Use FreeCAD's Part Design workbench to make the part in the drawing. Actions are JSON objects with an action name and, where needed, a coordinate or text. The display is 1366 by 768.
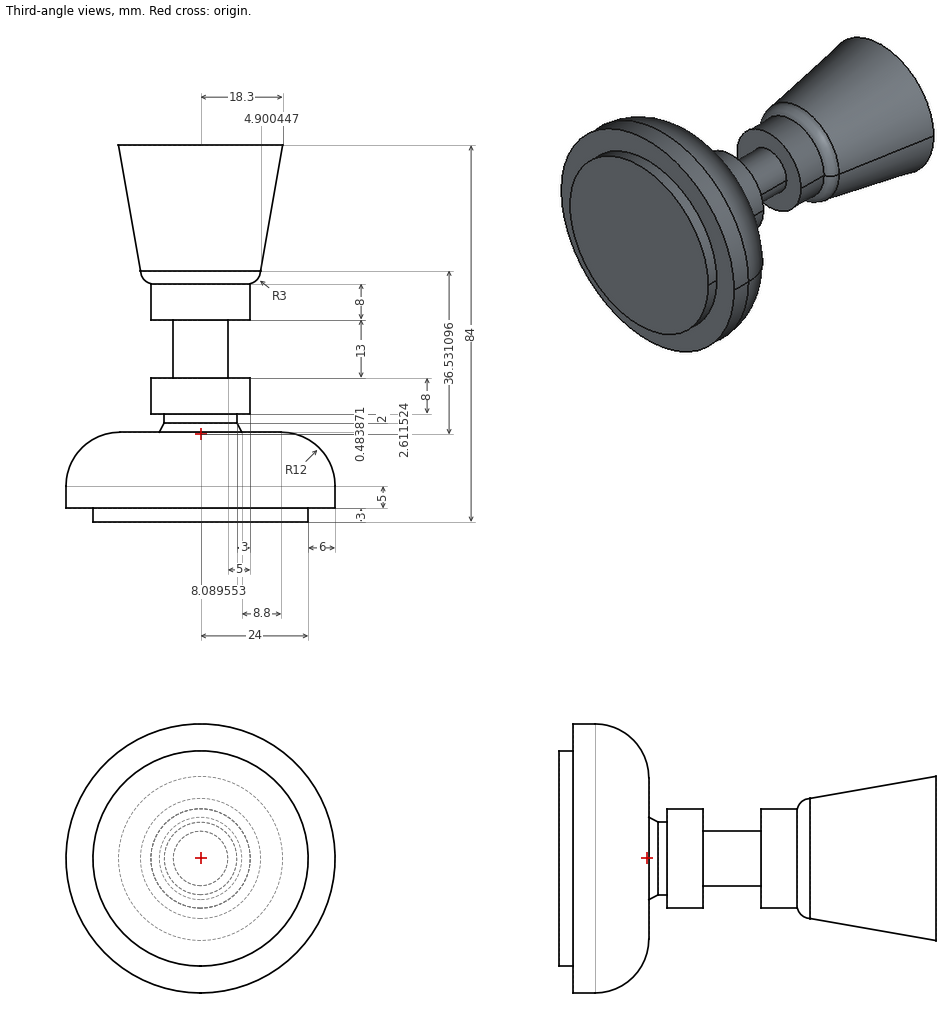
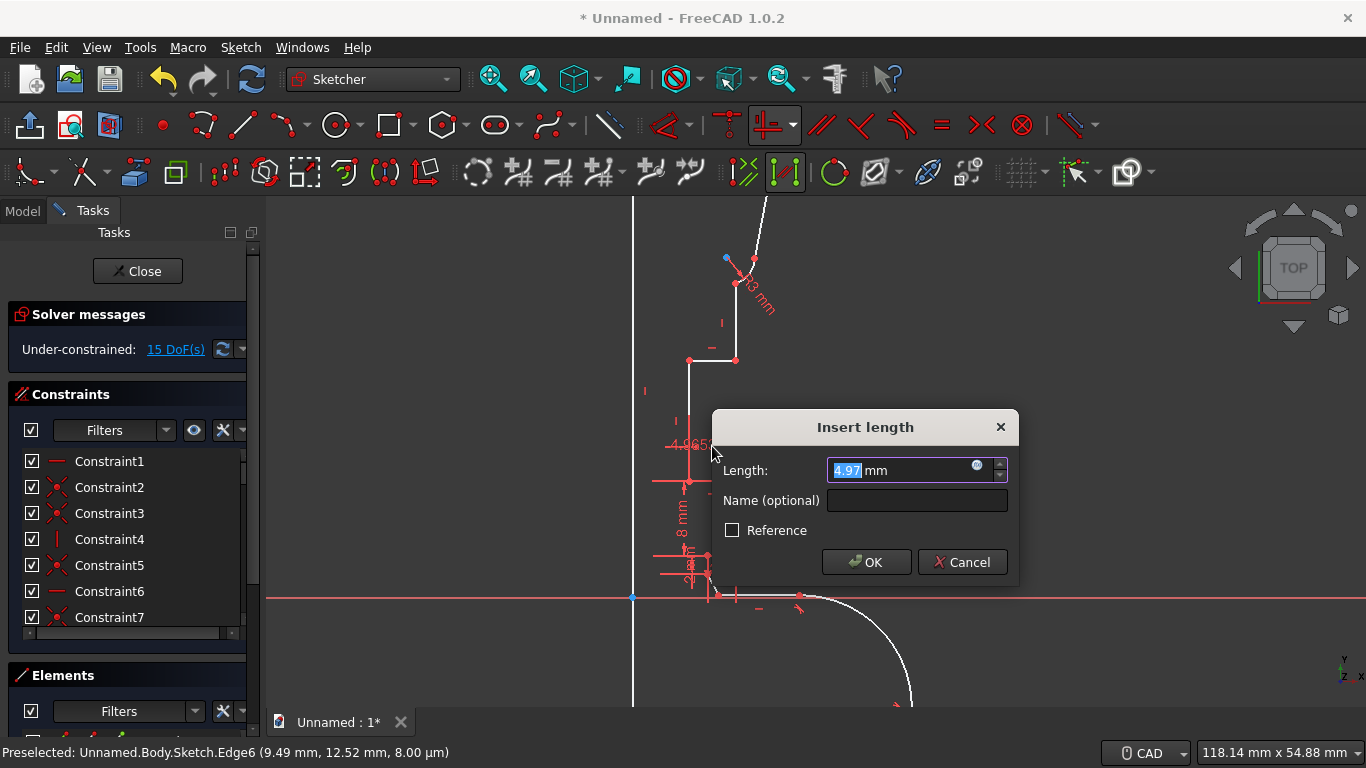
{"action": "type", "text": "5"}
{"action": "key", "text": "Return"}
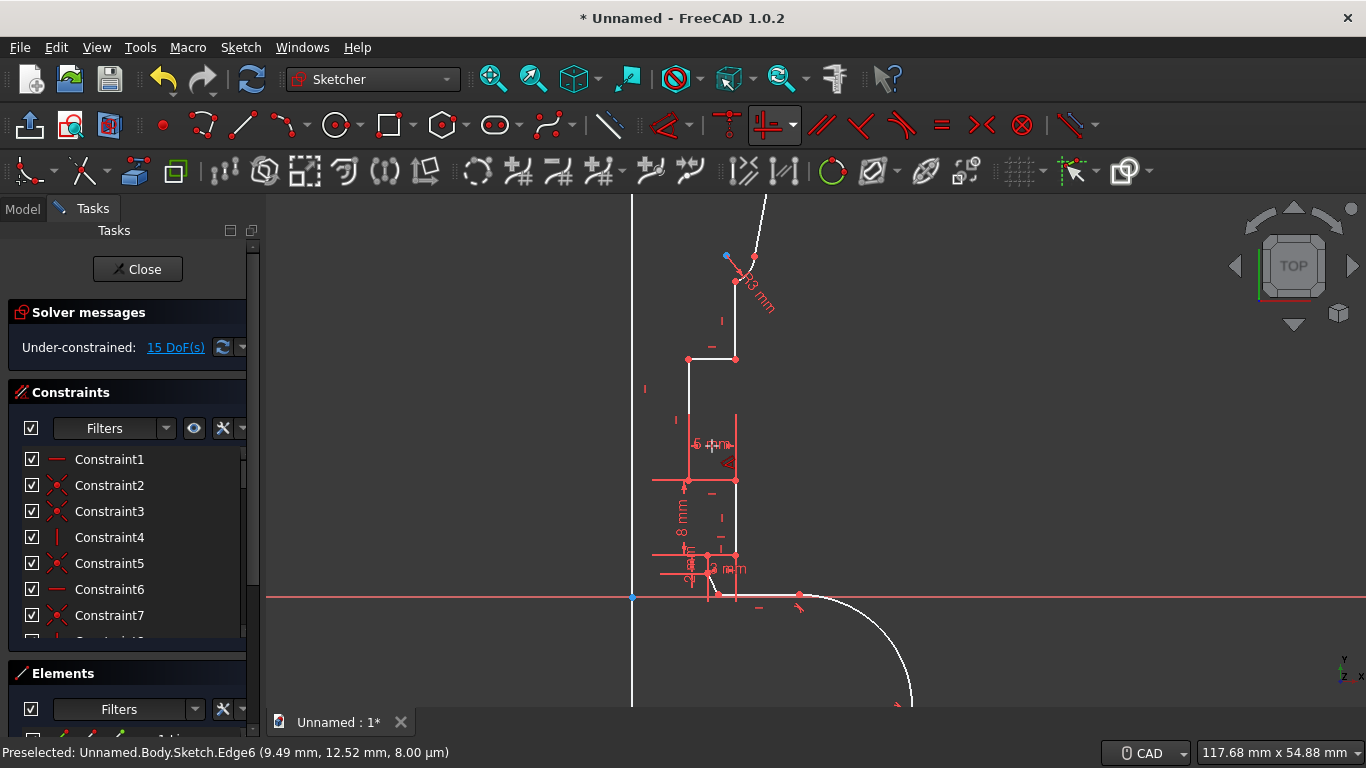
{"action": "left_click", "coordinate": [703, 359]}
{"action": "left_click", "coordinate": [712, 325]}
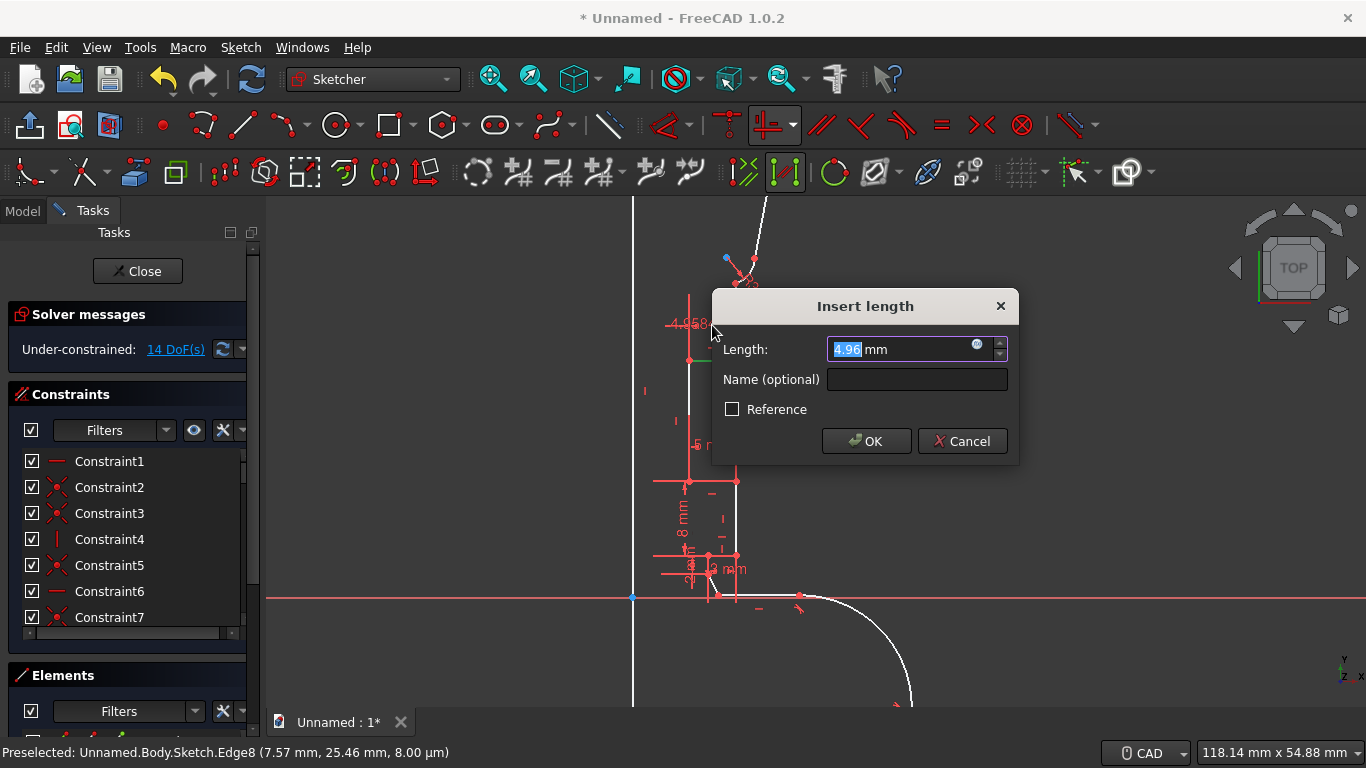
{"action": "type", "text": "5"}
{"action": "key", "text": "Return"}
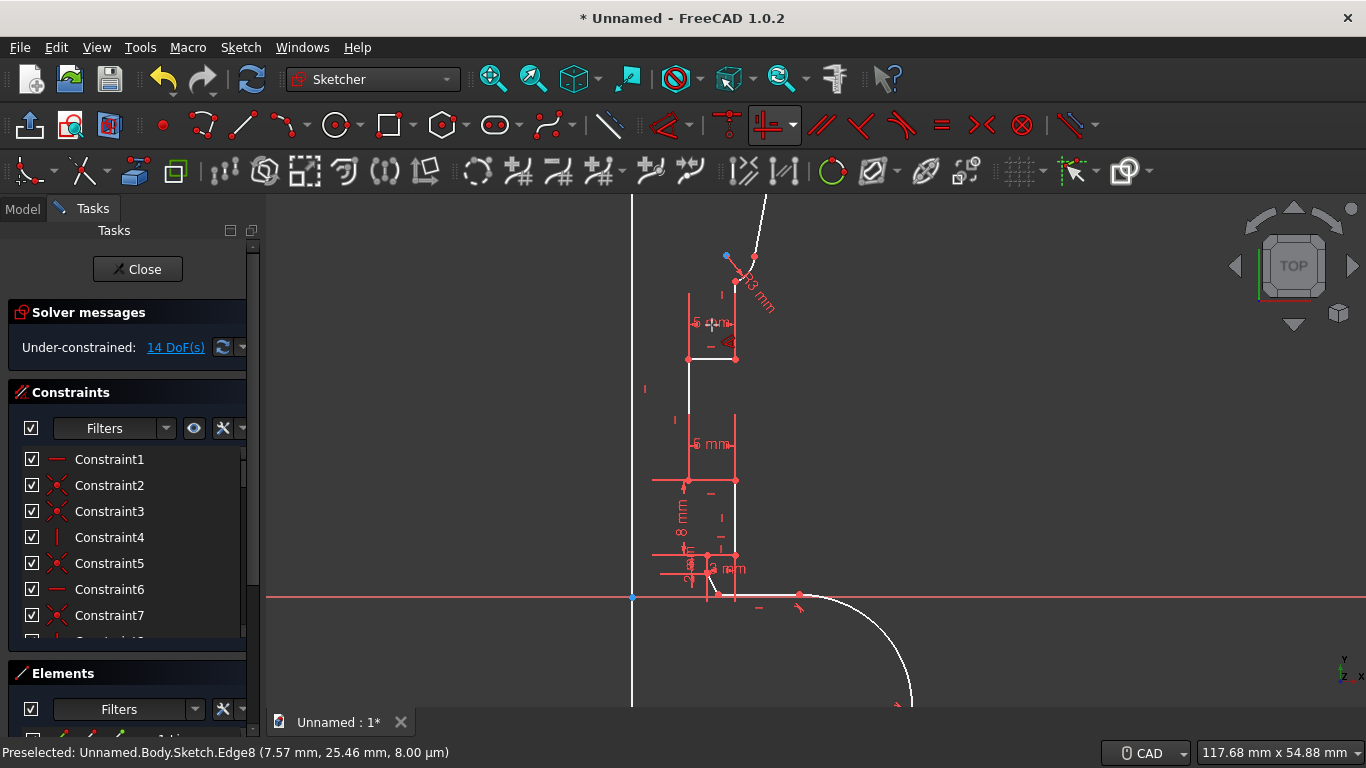
{"action": "left_click", "coordinate": [735, 336]}
{"action": "left_click", "coordinate": [769, 348]}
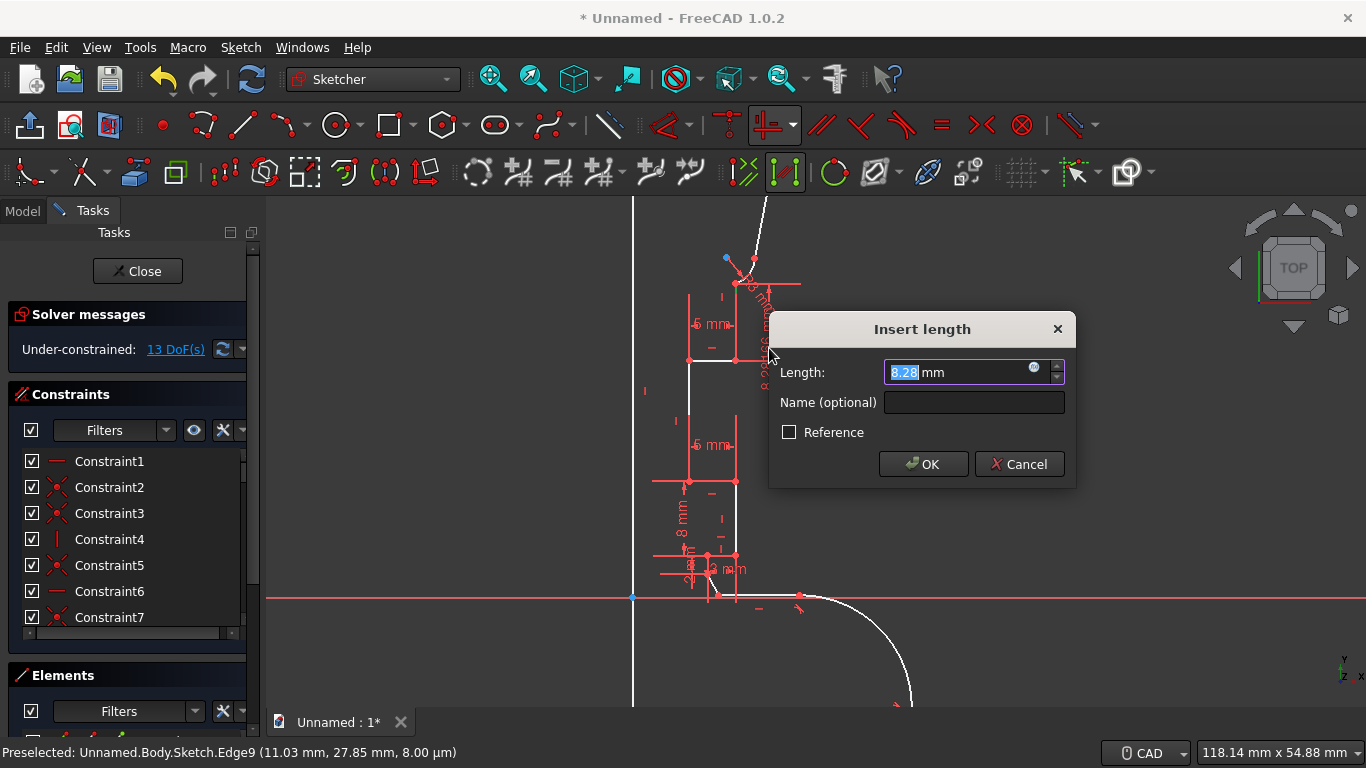
{"action": "type", "text": "8"}
{"action": "key", "text": "Return"}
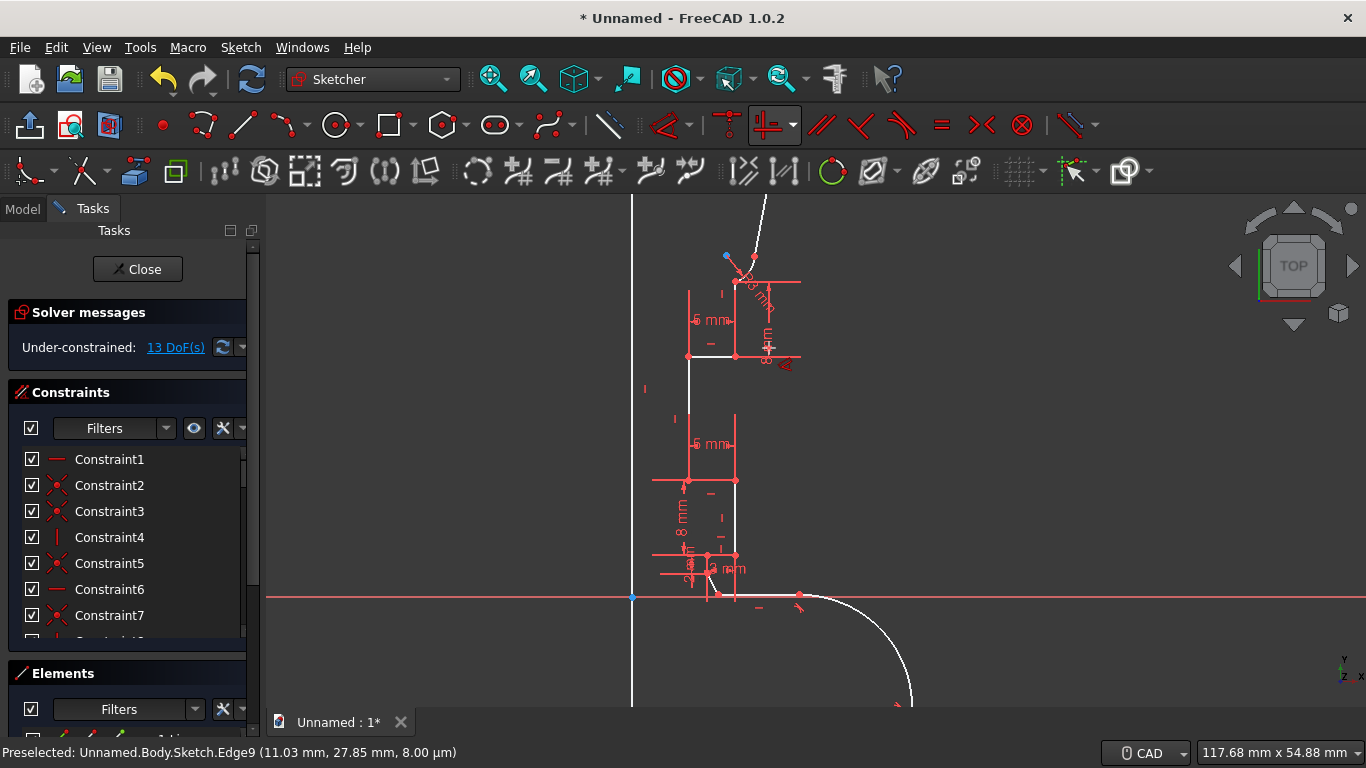
{"action": "scroll", "coordinate": [727, 502], "scroll_direction": "down", "scroll_amount": 4}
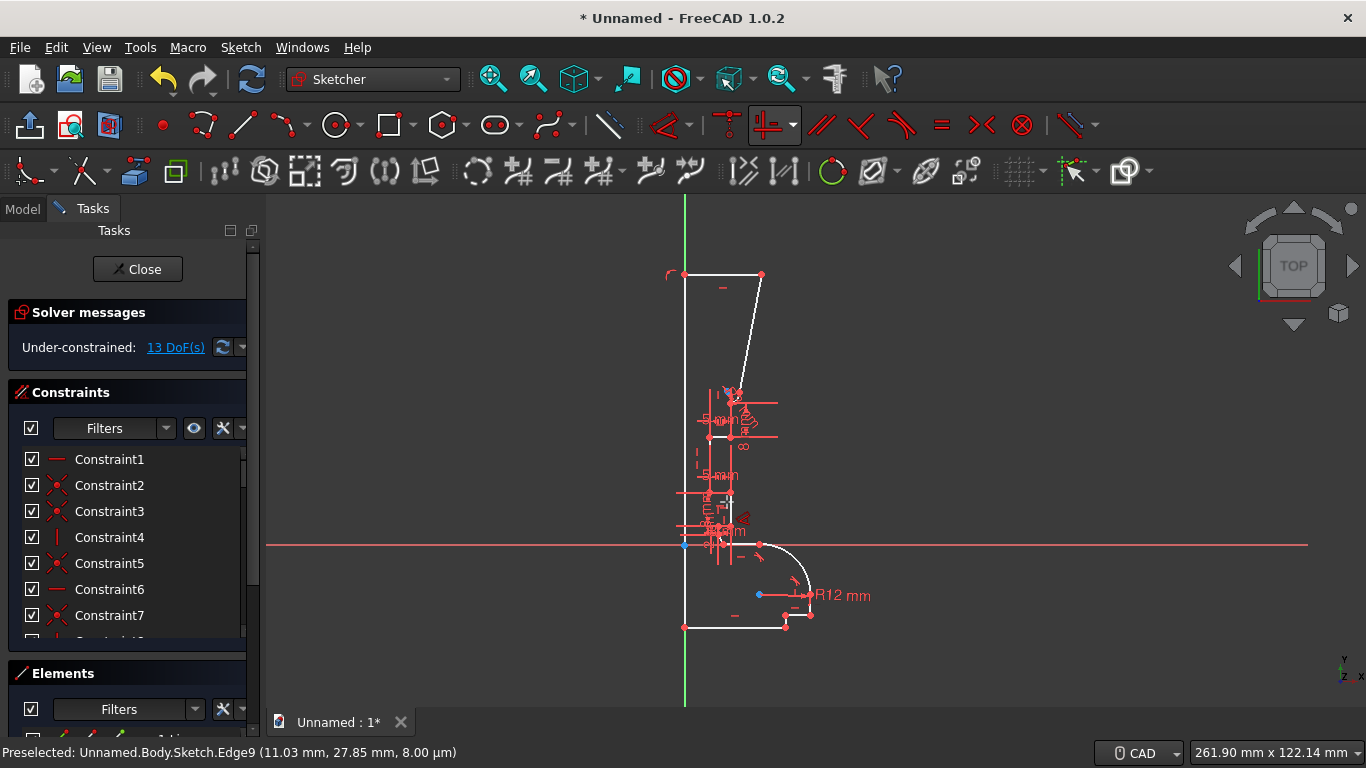
{"action": "scroll", "coordinate": [786, 623], "scroll_direction": "up", "scroll_amount": 6}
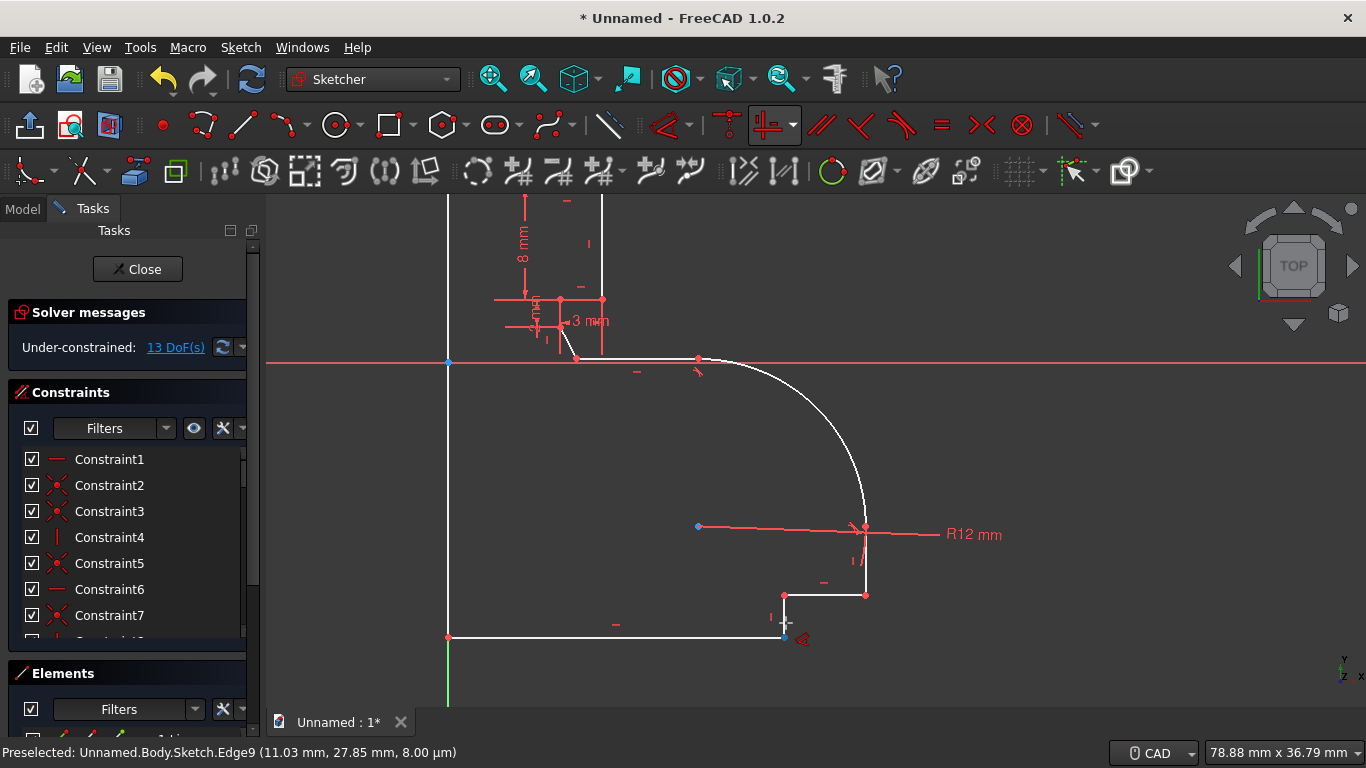
{"action": "left_click", "coordinate": [784, 621]}
{"action": "left_click", "coordinate": [818, 616]}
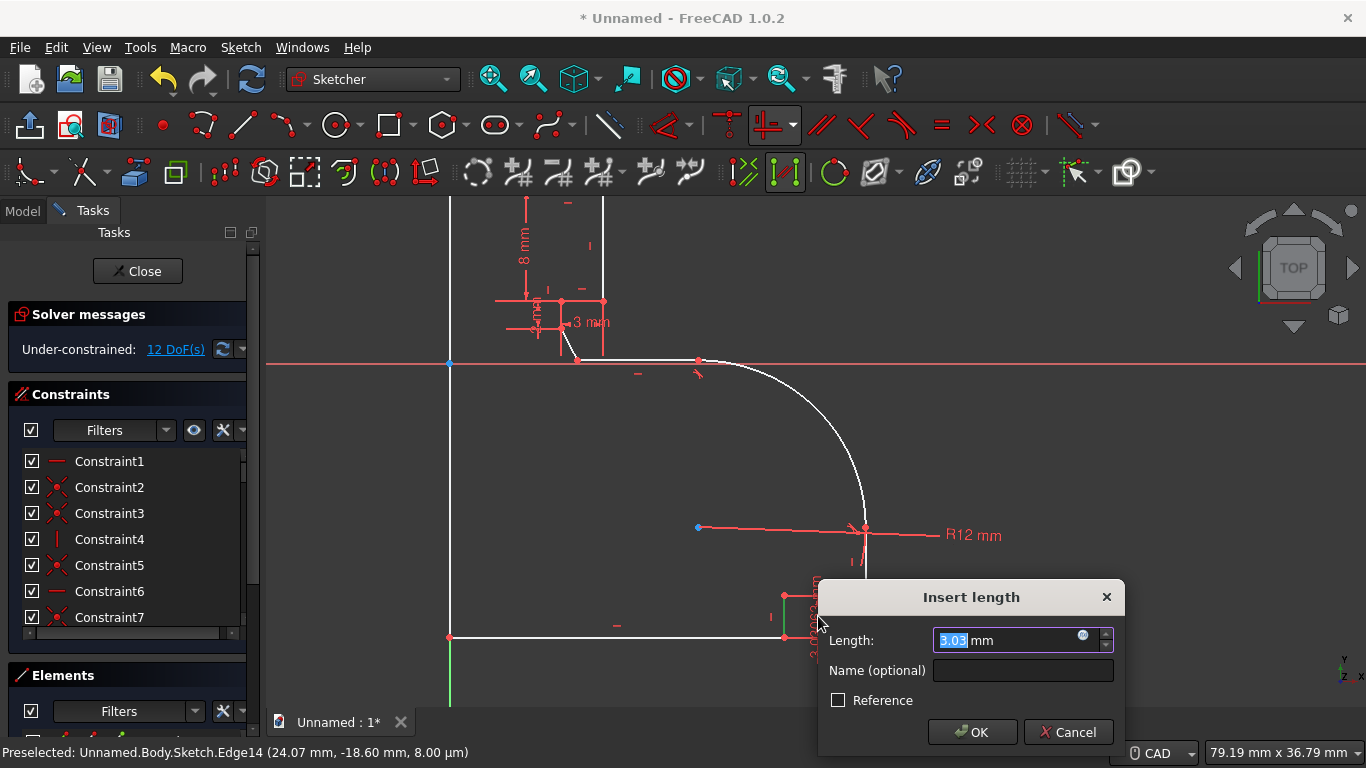
{"action": "type", "text": "3"}
{"action": "key", "text": "Return"}